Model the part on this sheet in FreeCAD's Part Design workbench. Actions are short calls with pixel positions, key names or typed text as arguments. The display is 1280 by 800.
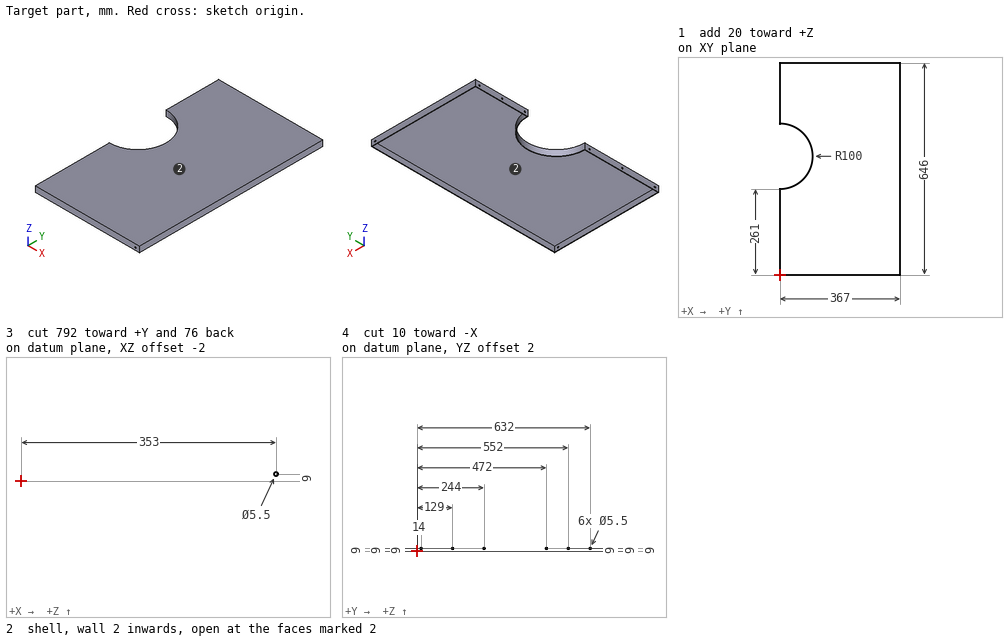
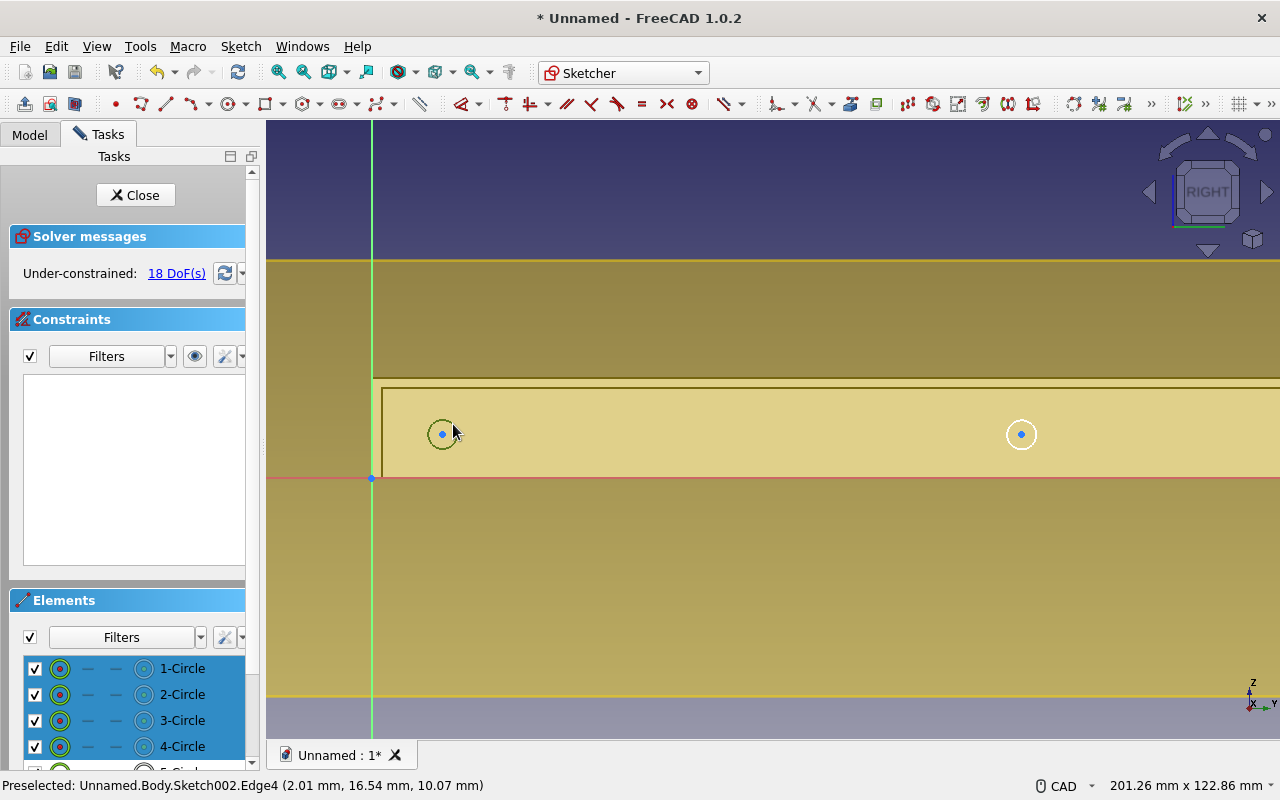
click(1032, 425)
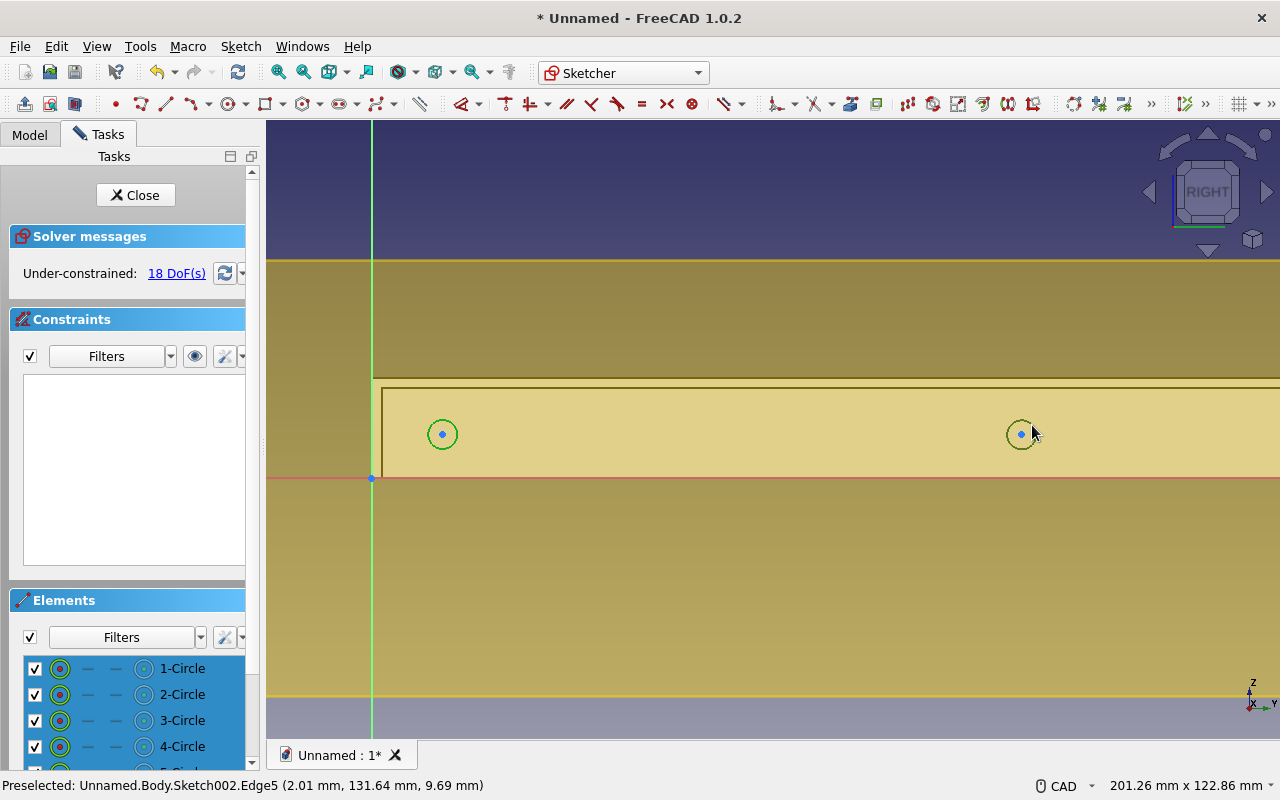
scroll(454, 426, down, 9)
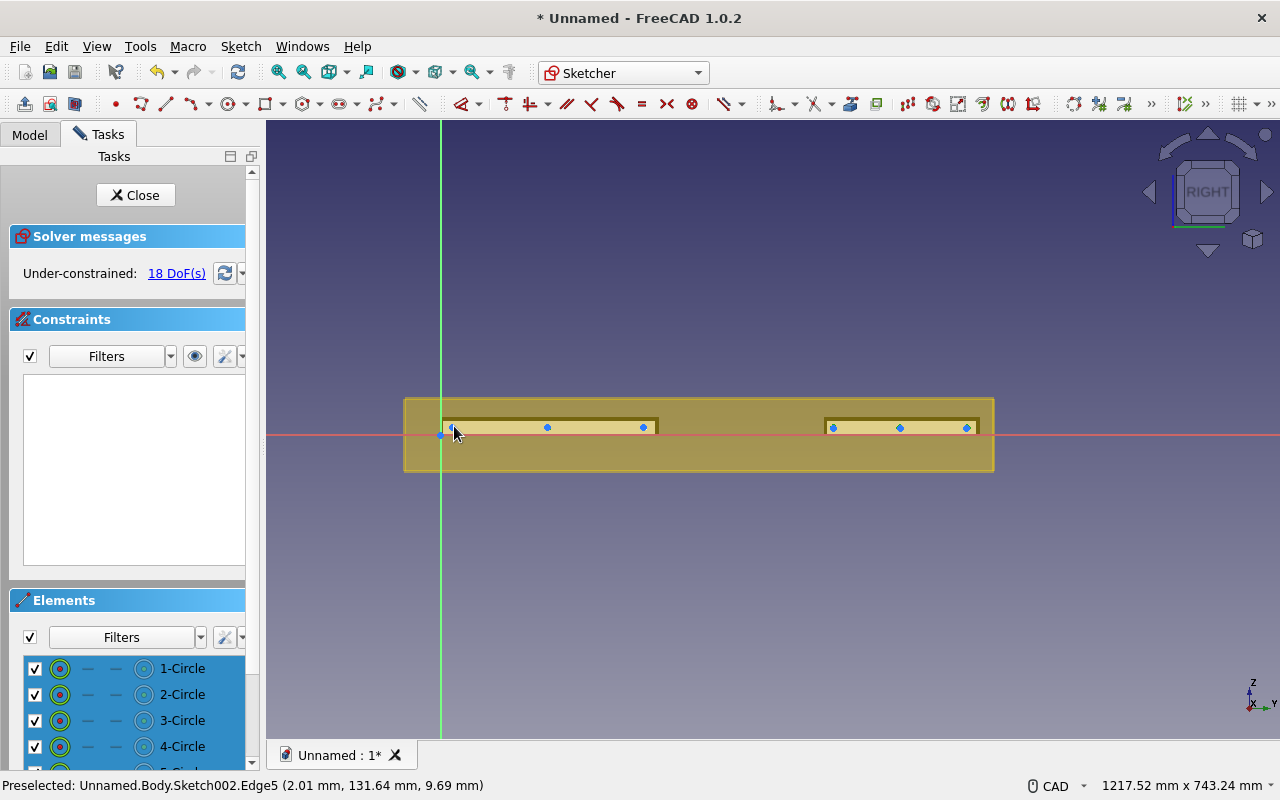
scroll(646, 426, up, 9)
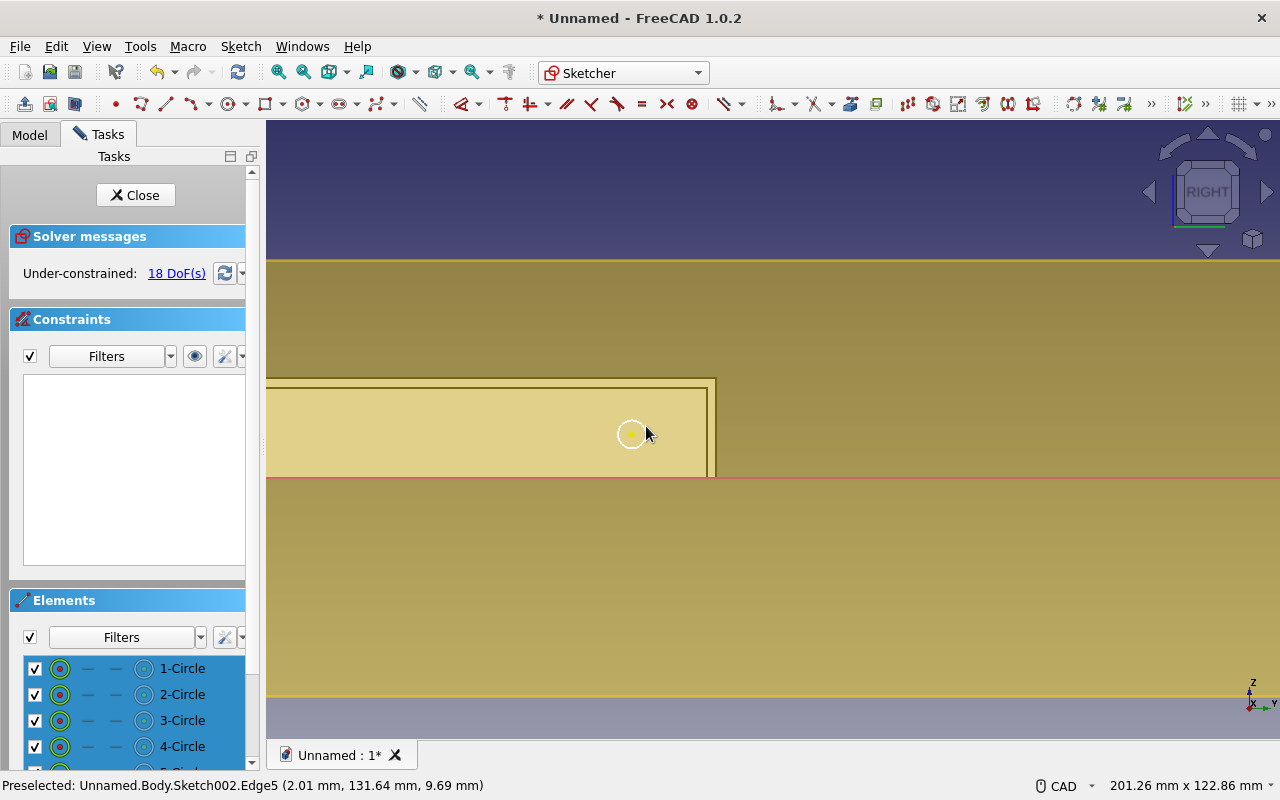
click(642, 425)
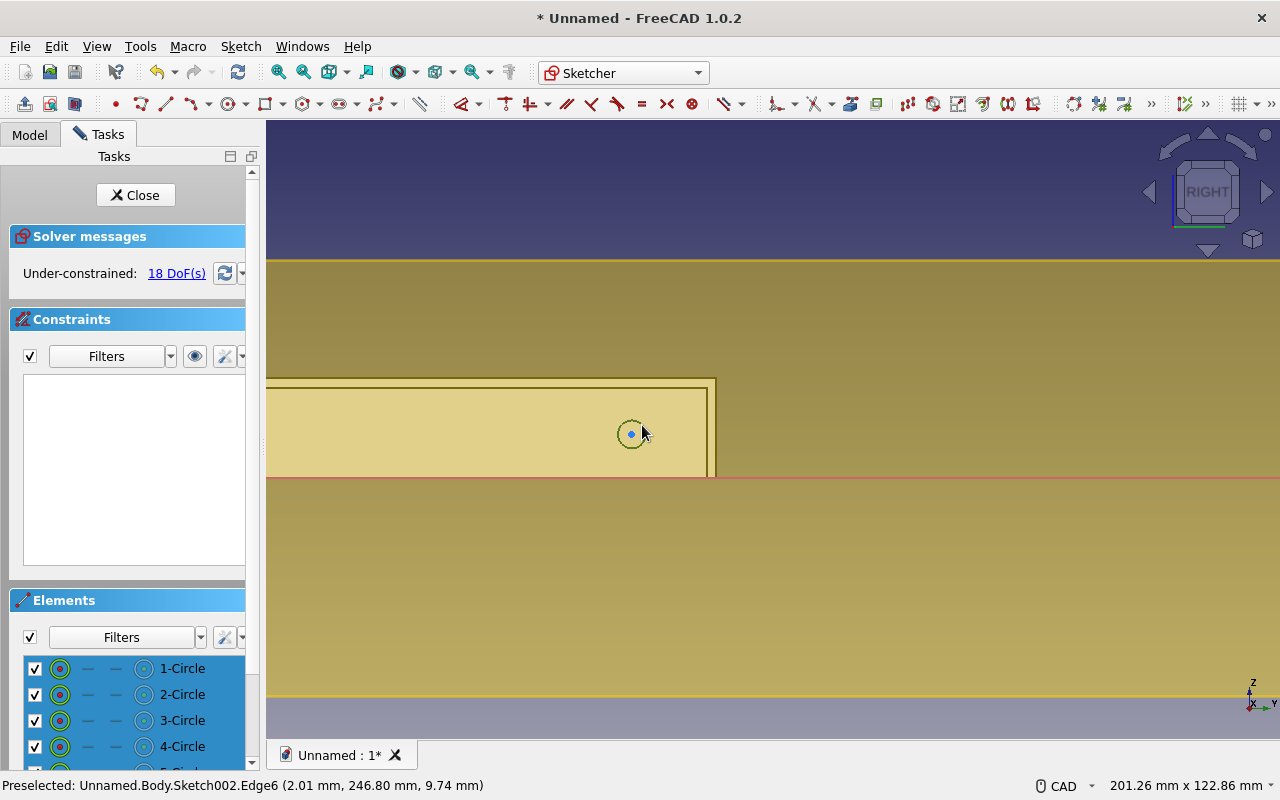
click(642, 104)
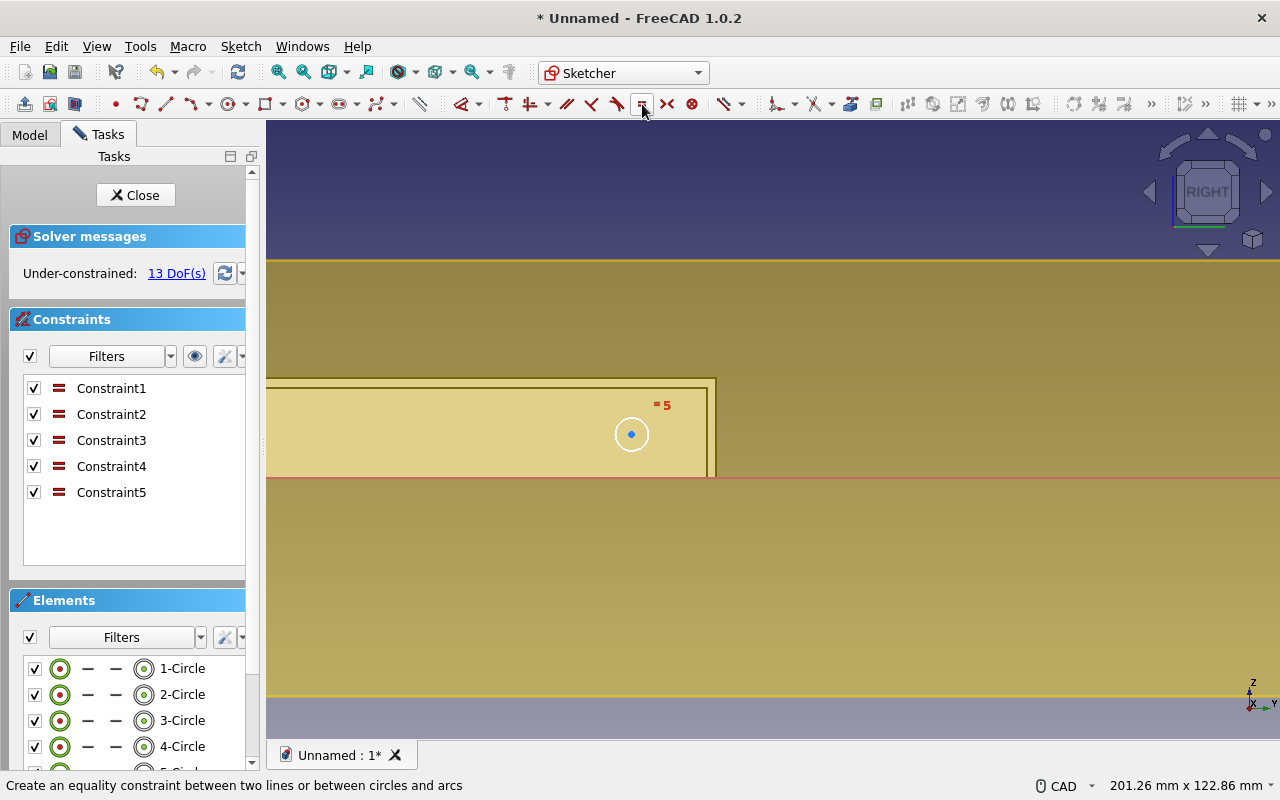
click(460, 104)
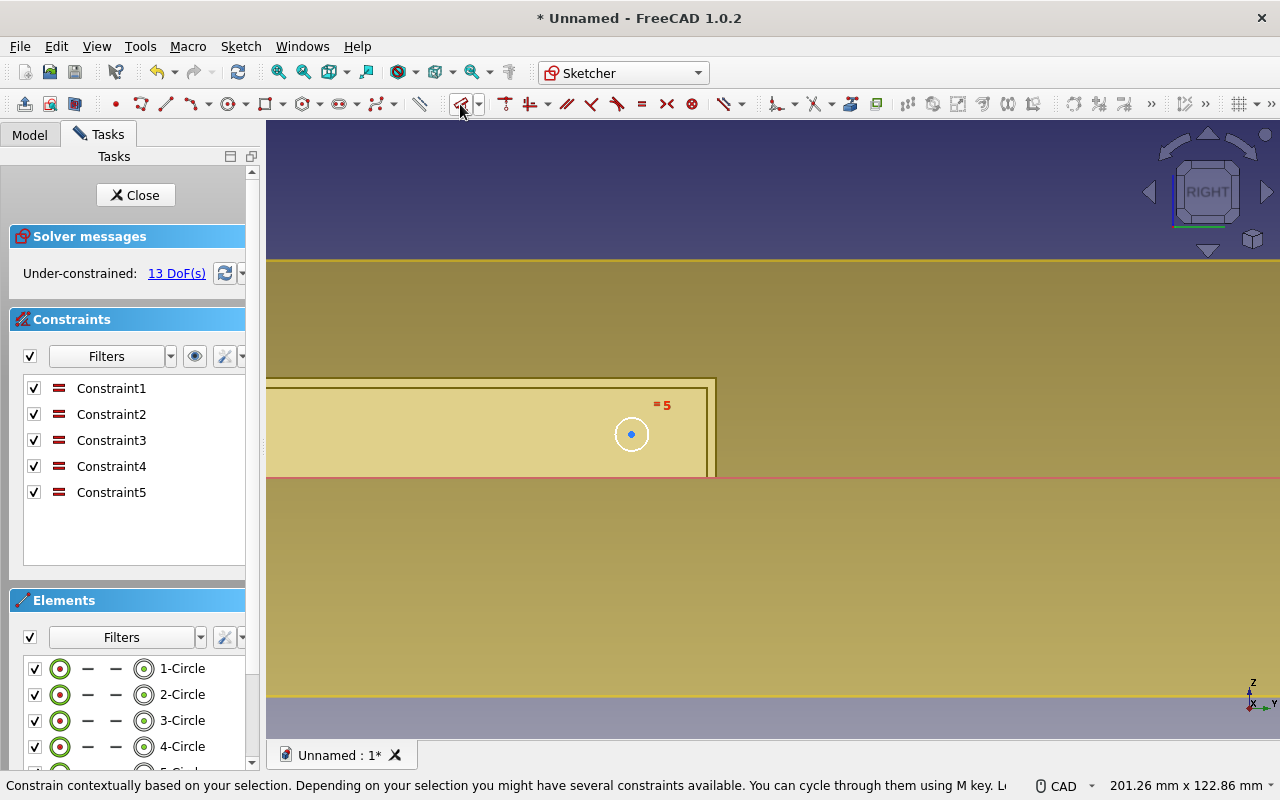
scroll(646, 426, down, 9)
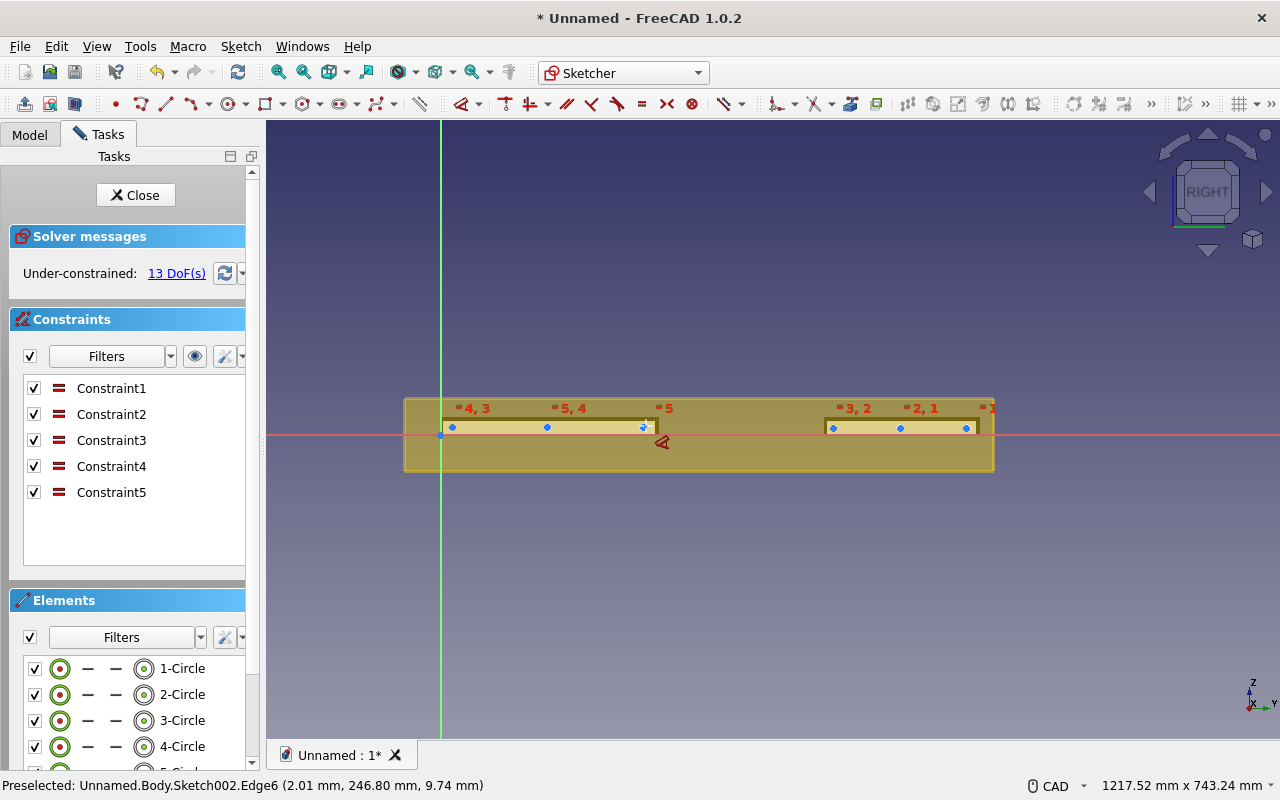
scroll(969, 426, up, 11)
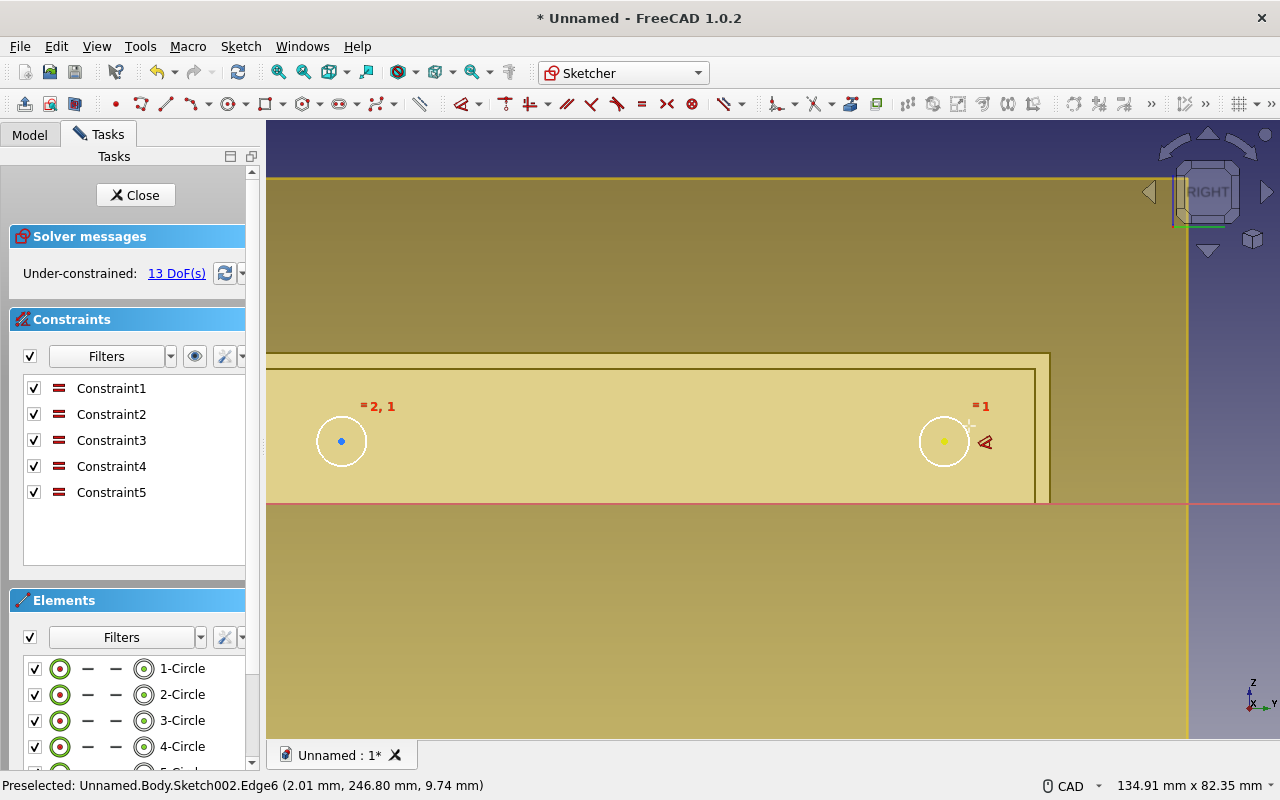
click(962, 424)
click(985, 401)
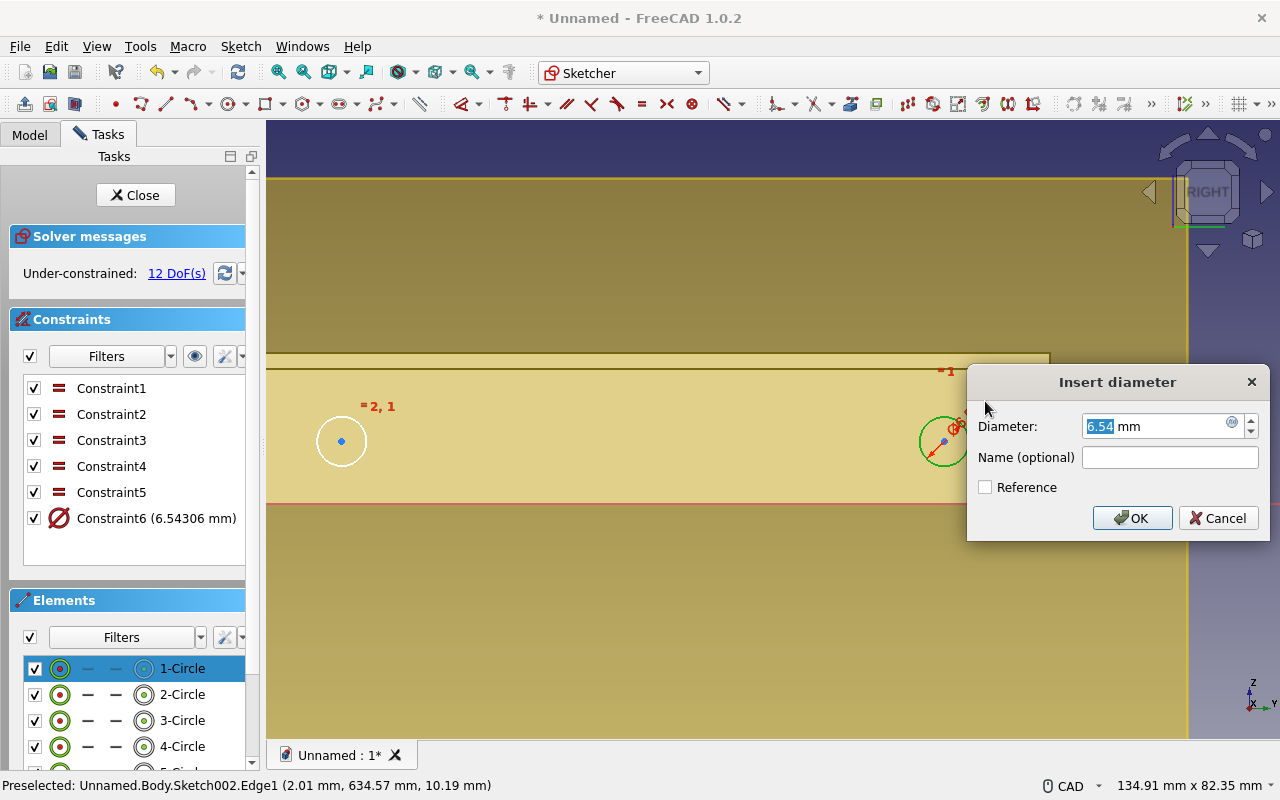
text(5.5)
key(Return)